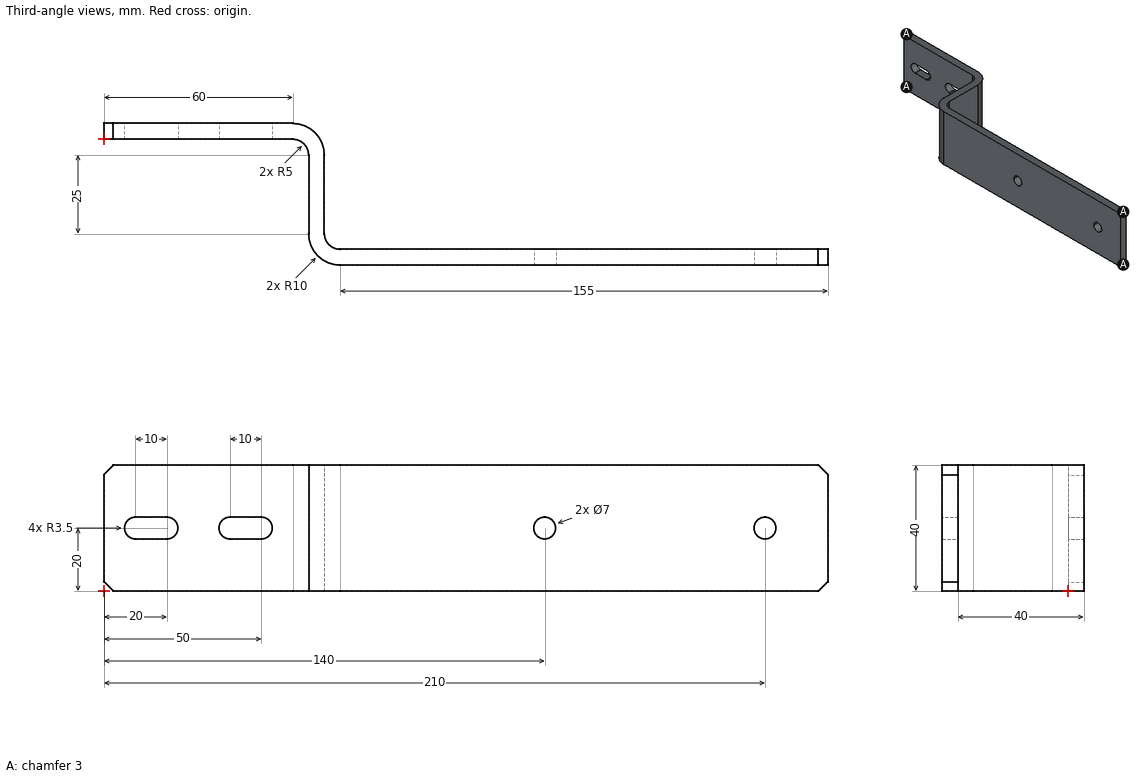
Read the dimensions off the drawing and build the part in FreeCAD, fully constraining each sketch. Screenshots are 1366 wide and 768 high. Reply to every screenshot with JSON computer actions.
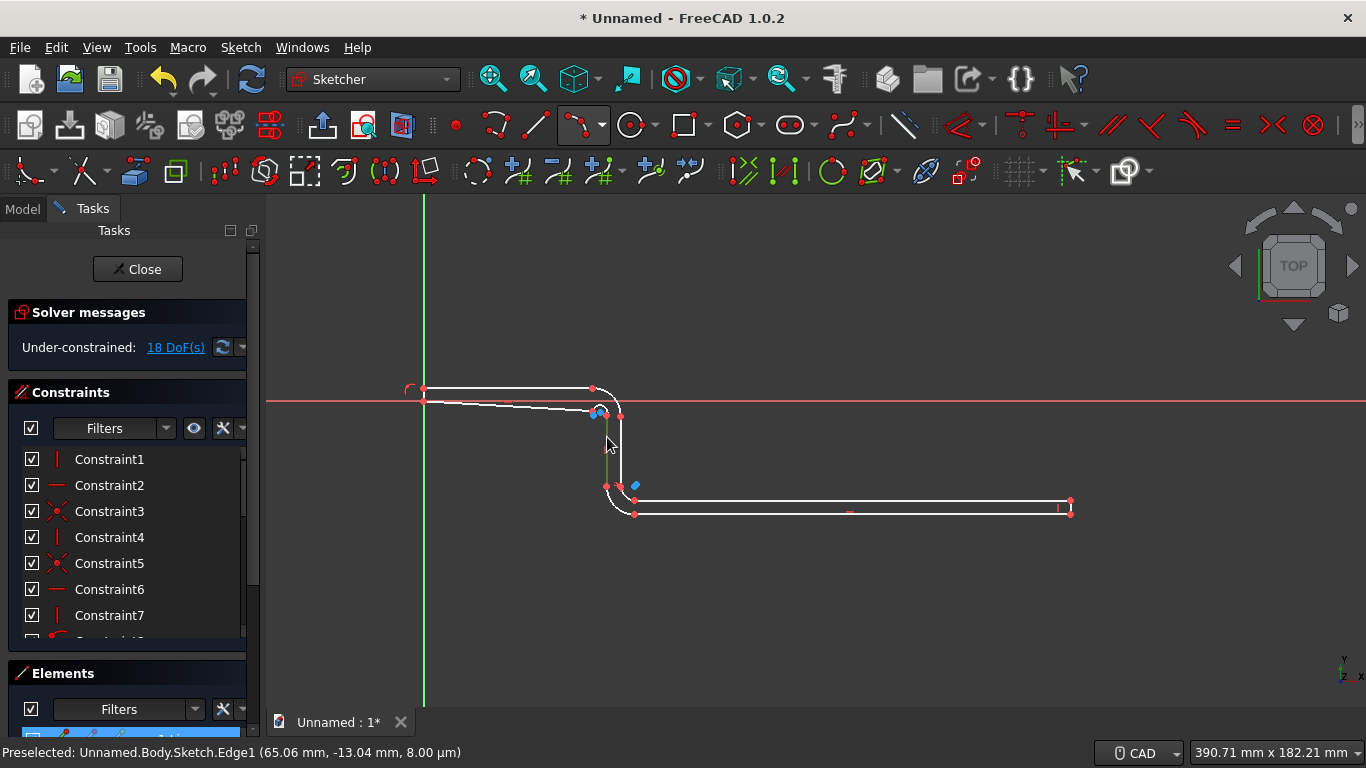
{"action": "scroll", "coordinate": [606, 409], "scroll_direction": "up", "scroll_amount": 4}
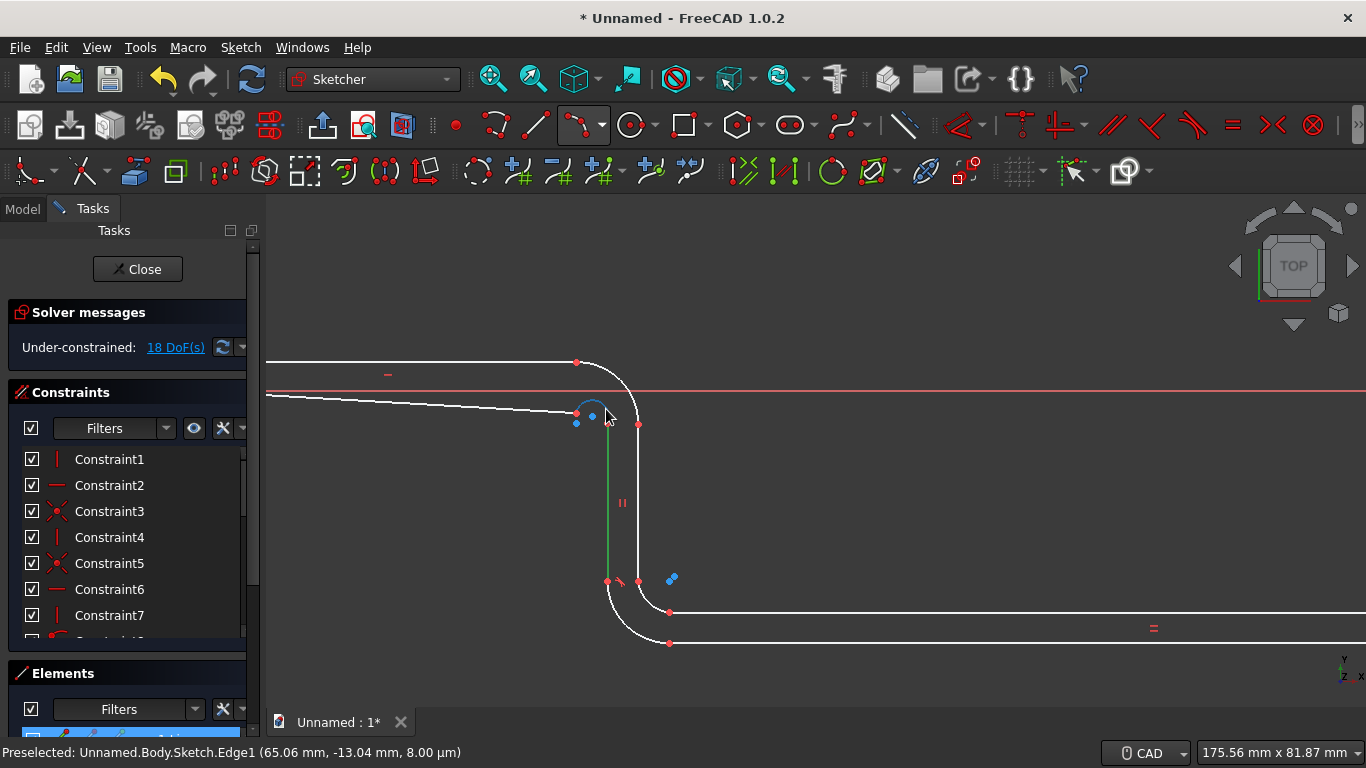
{"action": "left_click", "coordinate": [606, 408]}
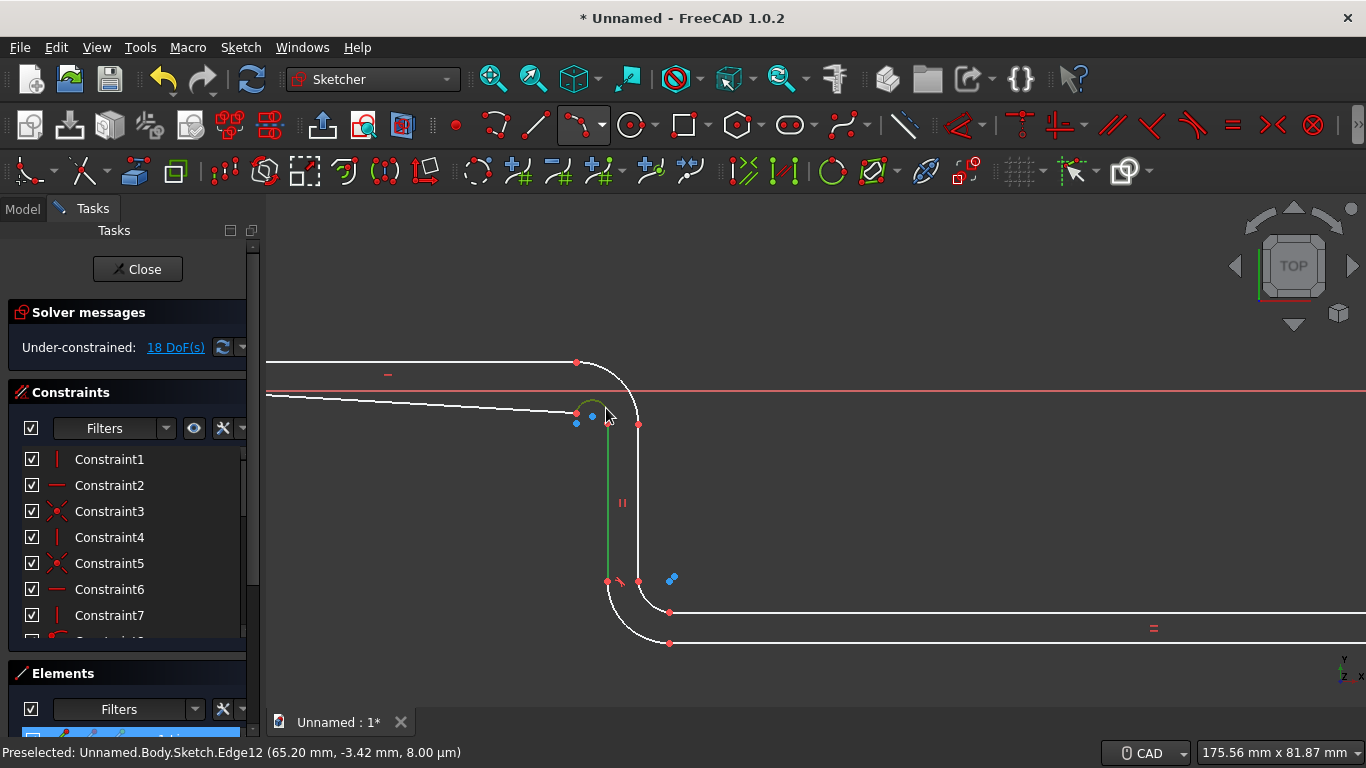
{"action": "left_click", "coordinate": [1194, 126]}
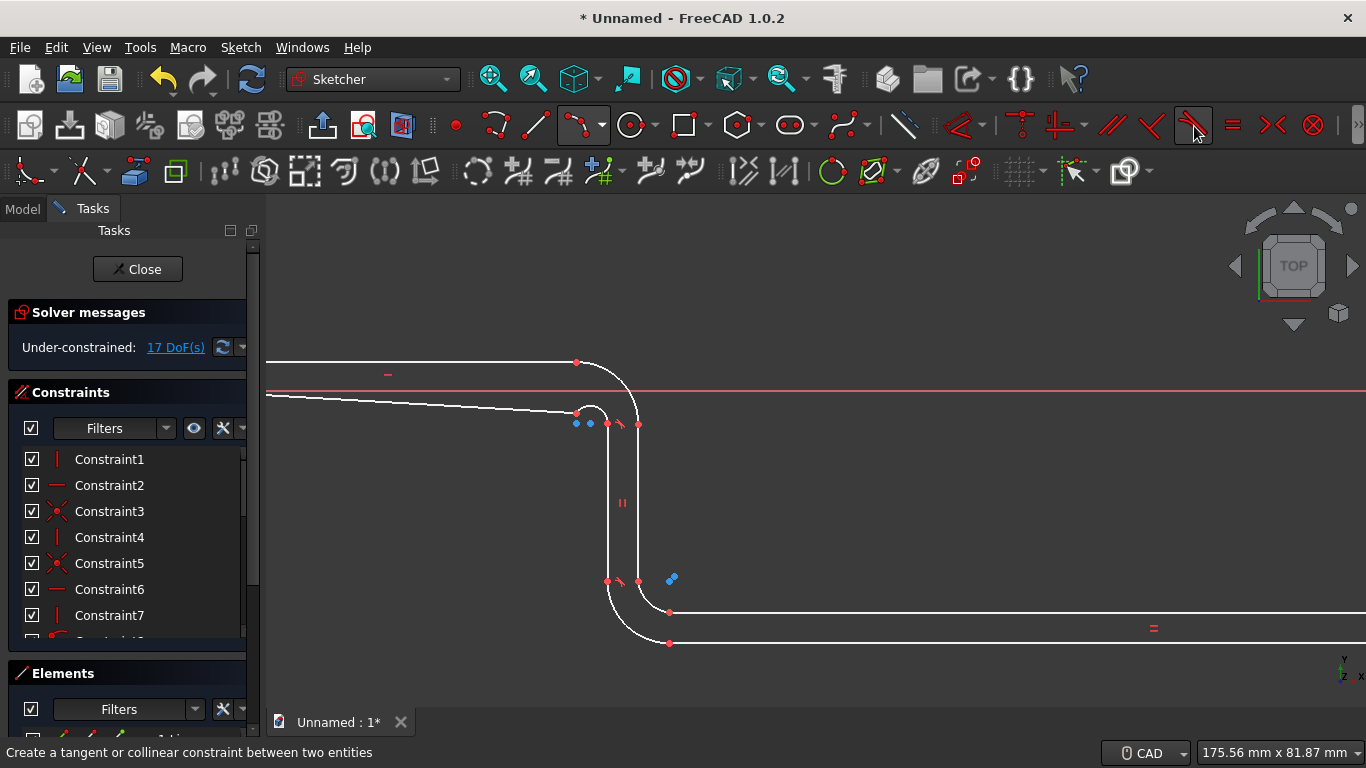
{"action": "left_click", "coordinate": [961, 643]}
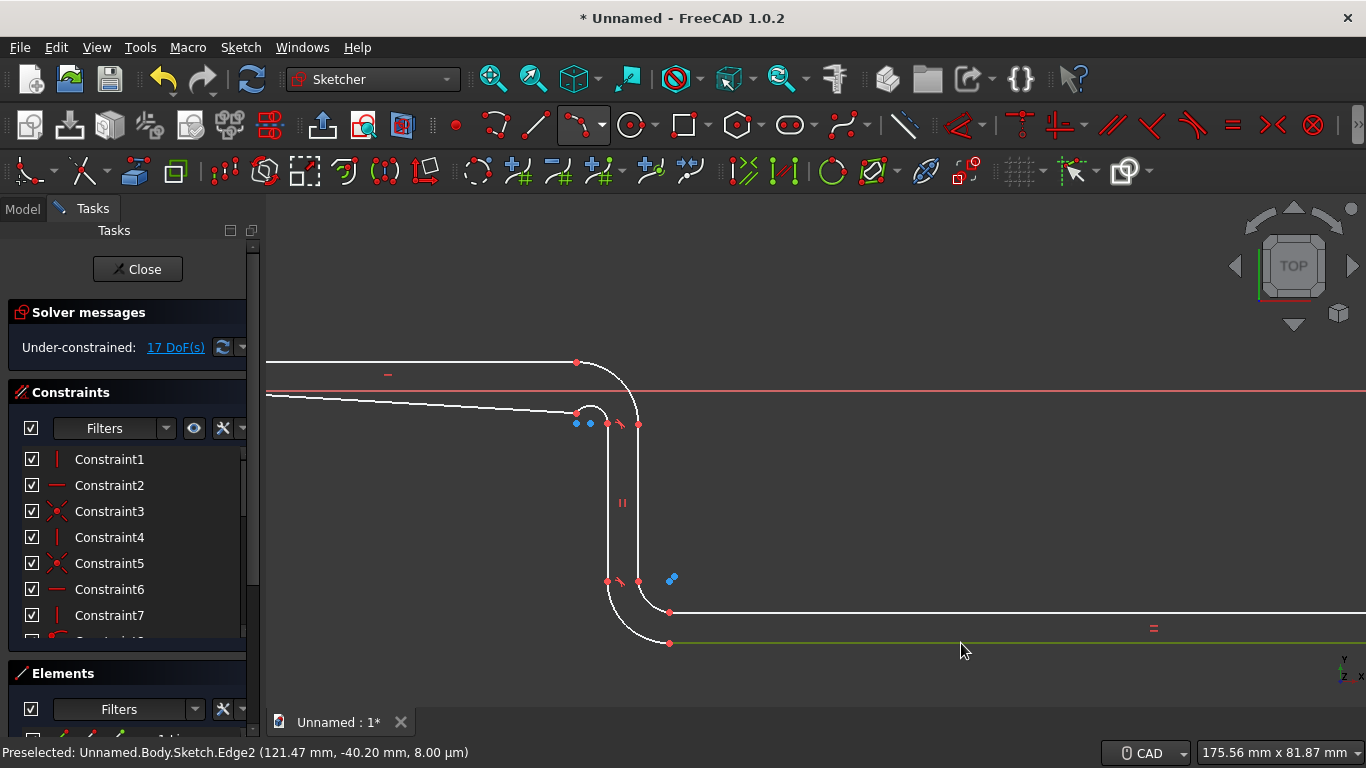
{"action": "left_click", "coordinate": [614, 609]}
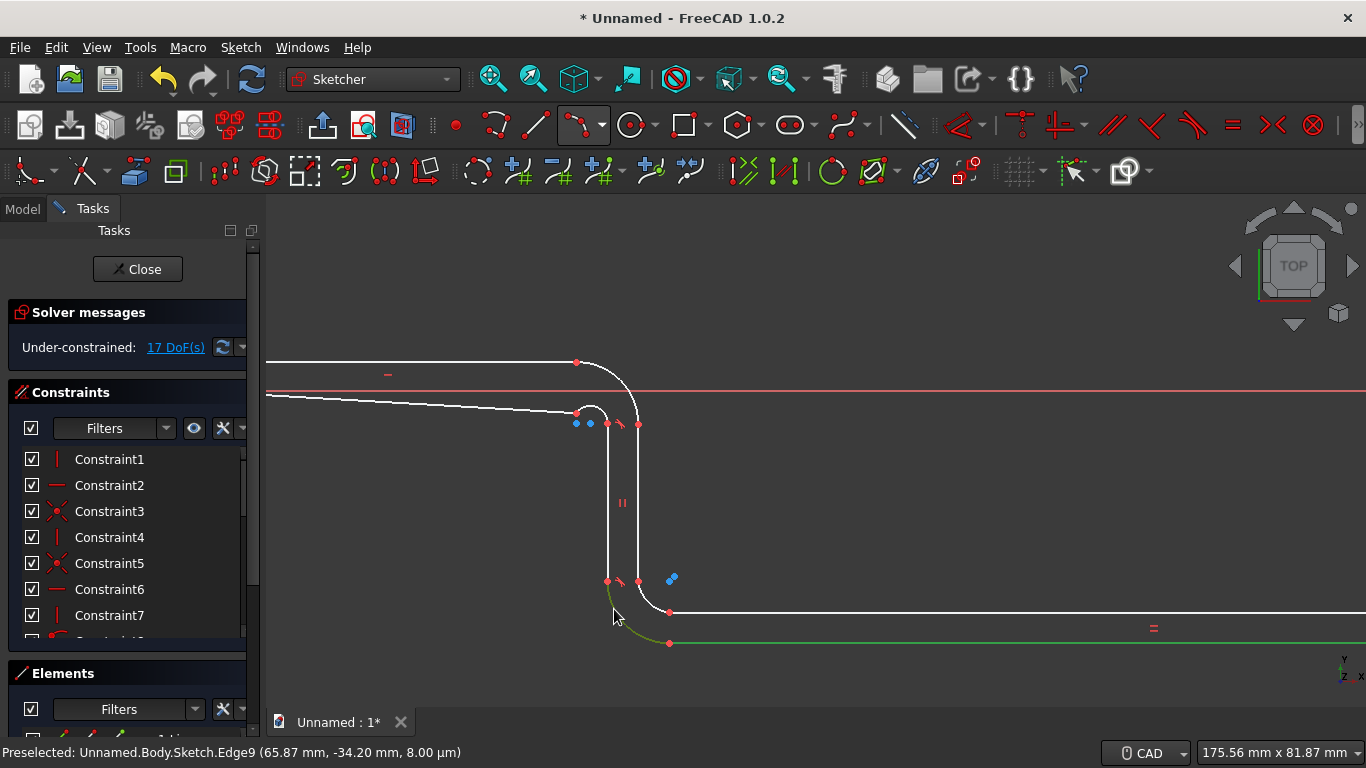
{"action": "left_click", "coordinate": [1194, 126]}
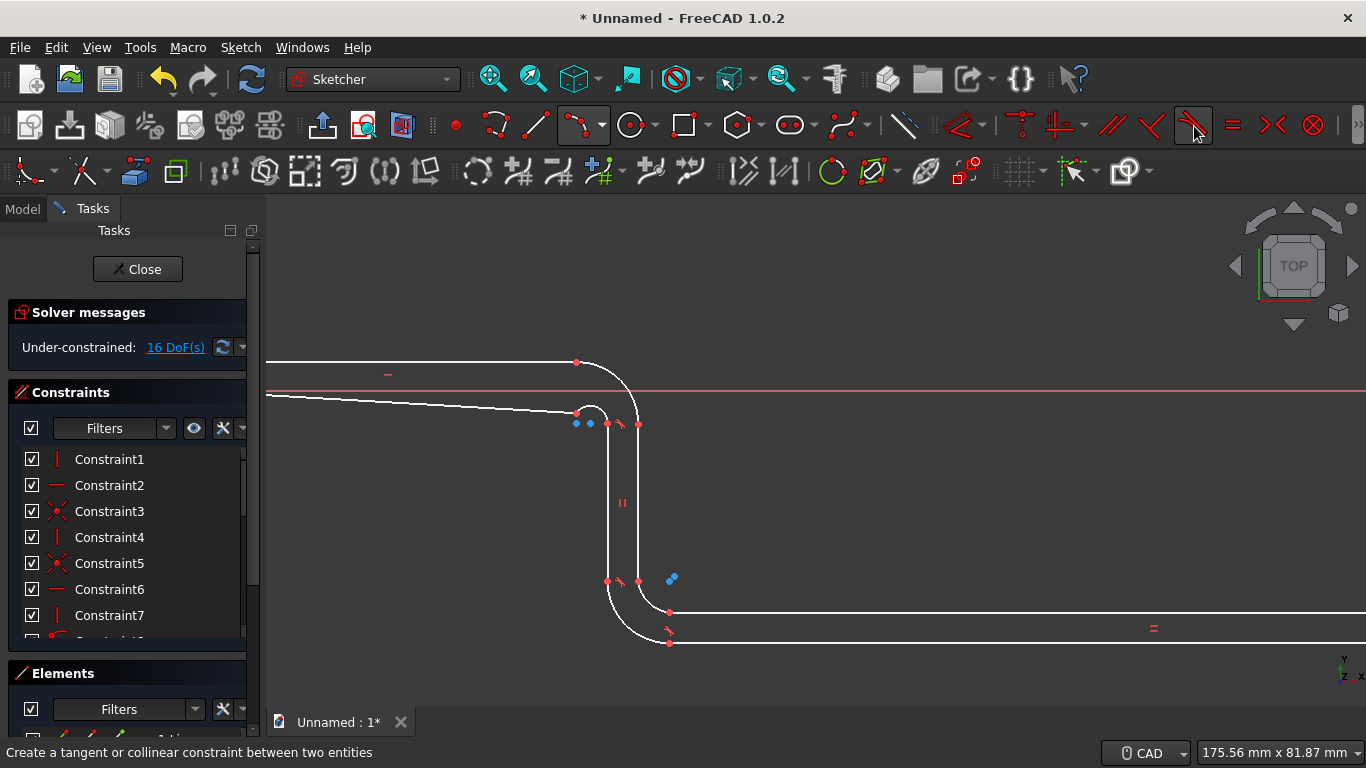
{"action": "left_click", "coordinate": [960, 613]}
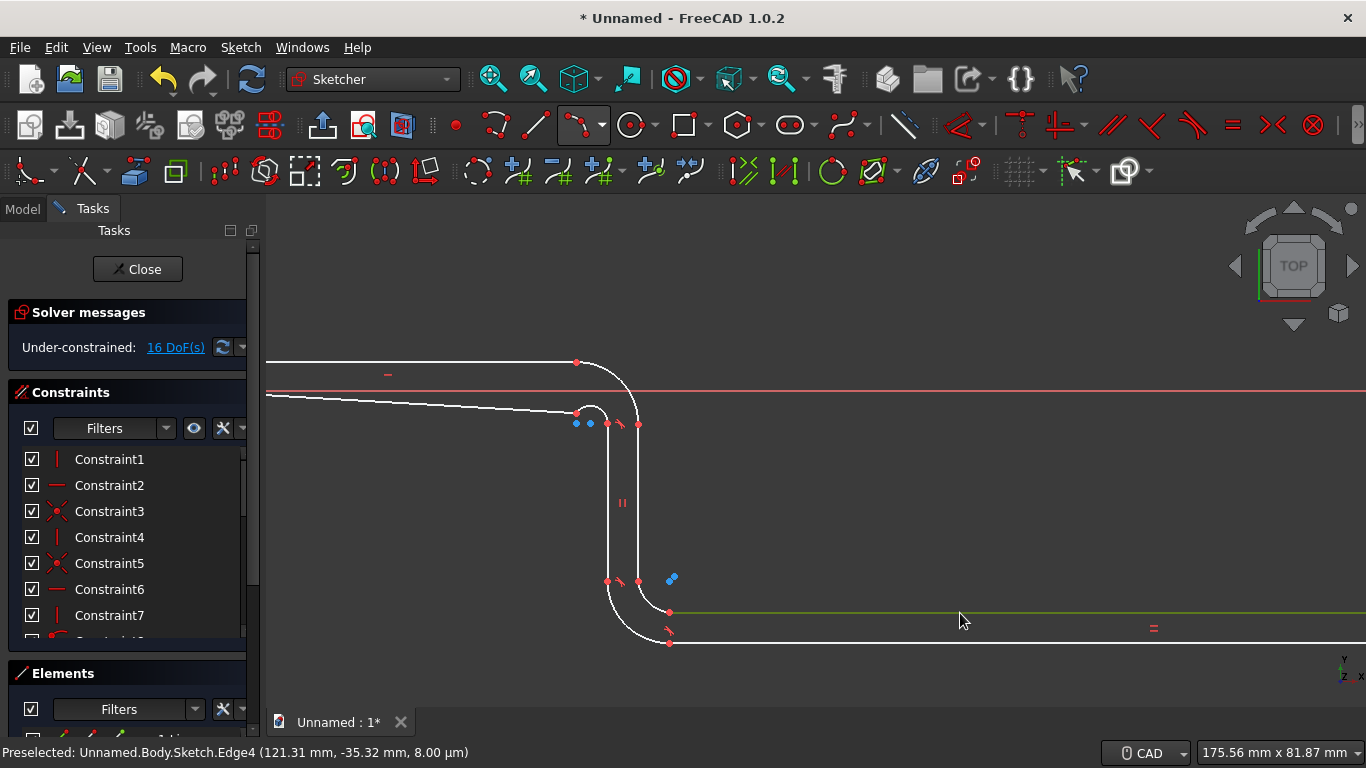
{"action": "left_click", "coordinate": [643, 595]}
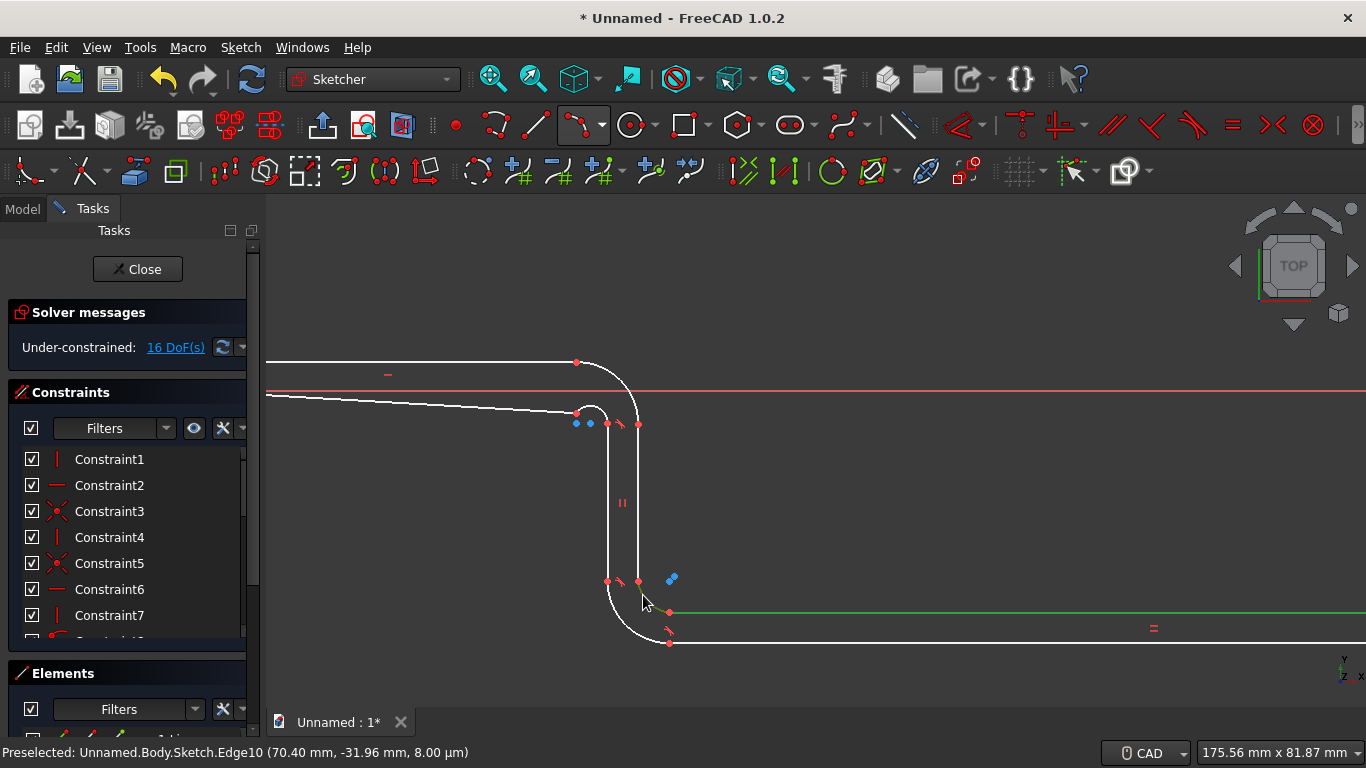
{"action": "left_click", "coordinate": [1194, 126]}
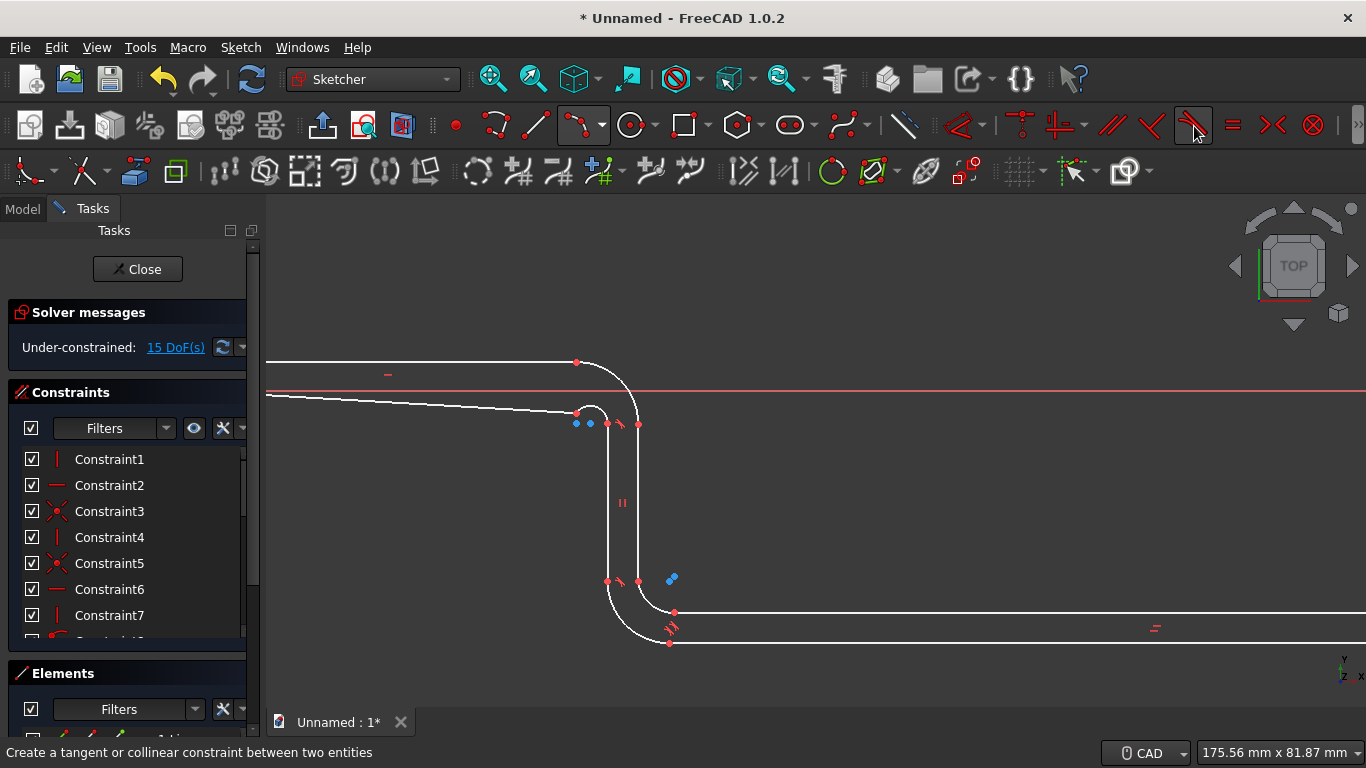
{"action": "left_click", "coordinate": [638, 534]}